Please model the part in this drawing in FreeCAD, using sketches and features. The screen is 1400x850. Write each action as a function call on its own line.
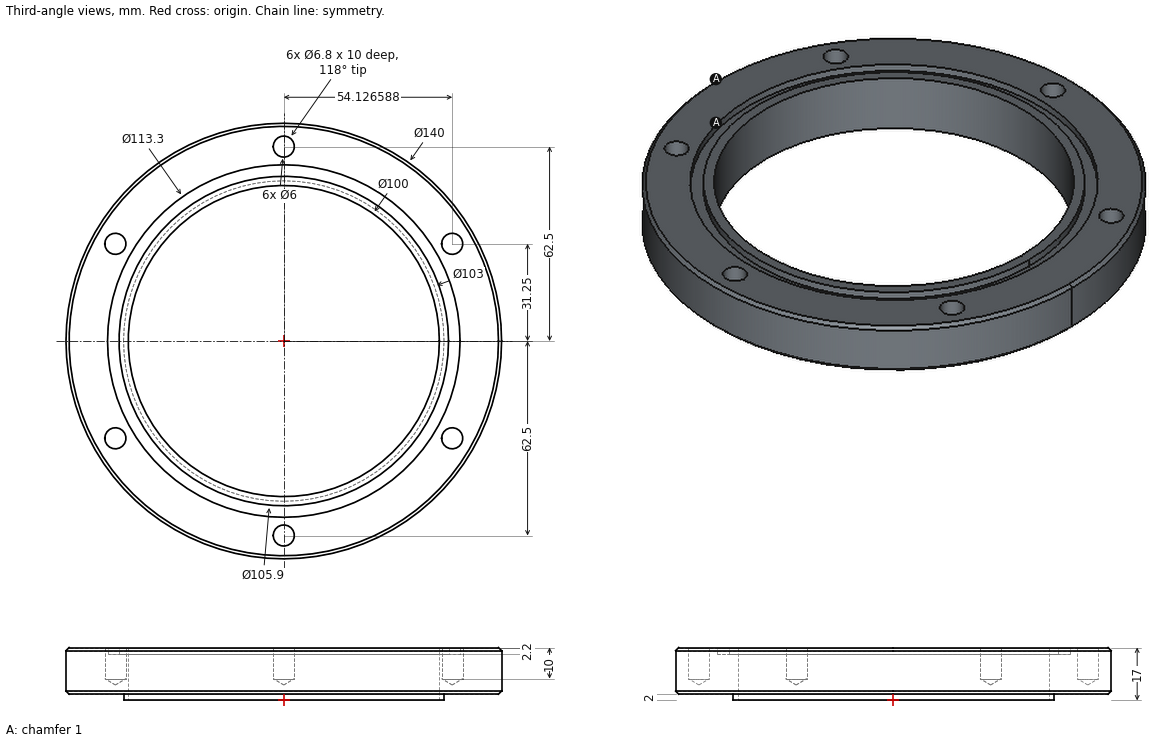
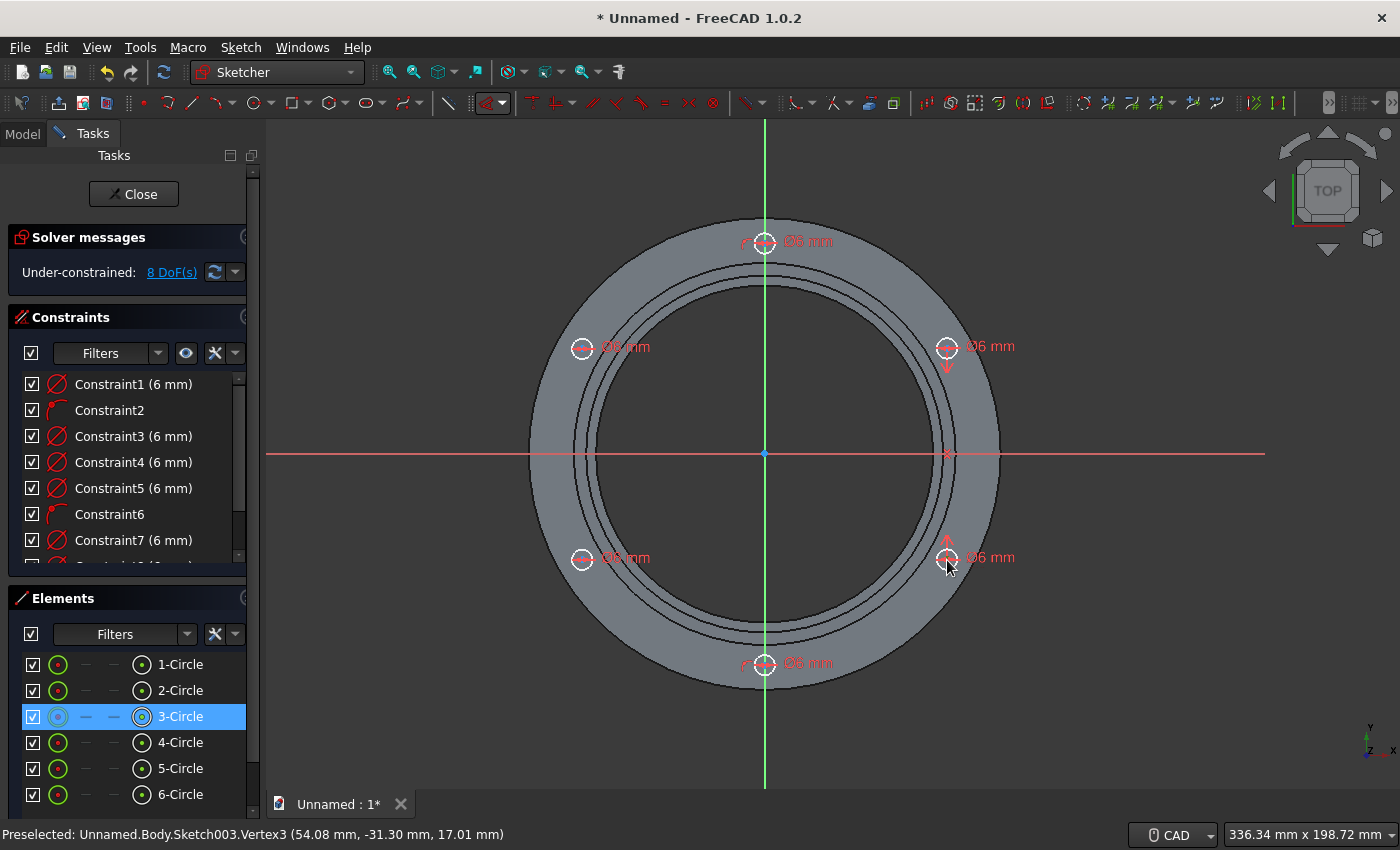
click(582, 560)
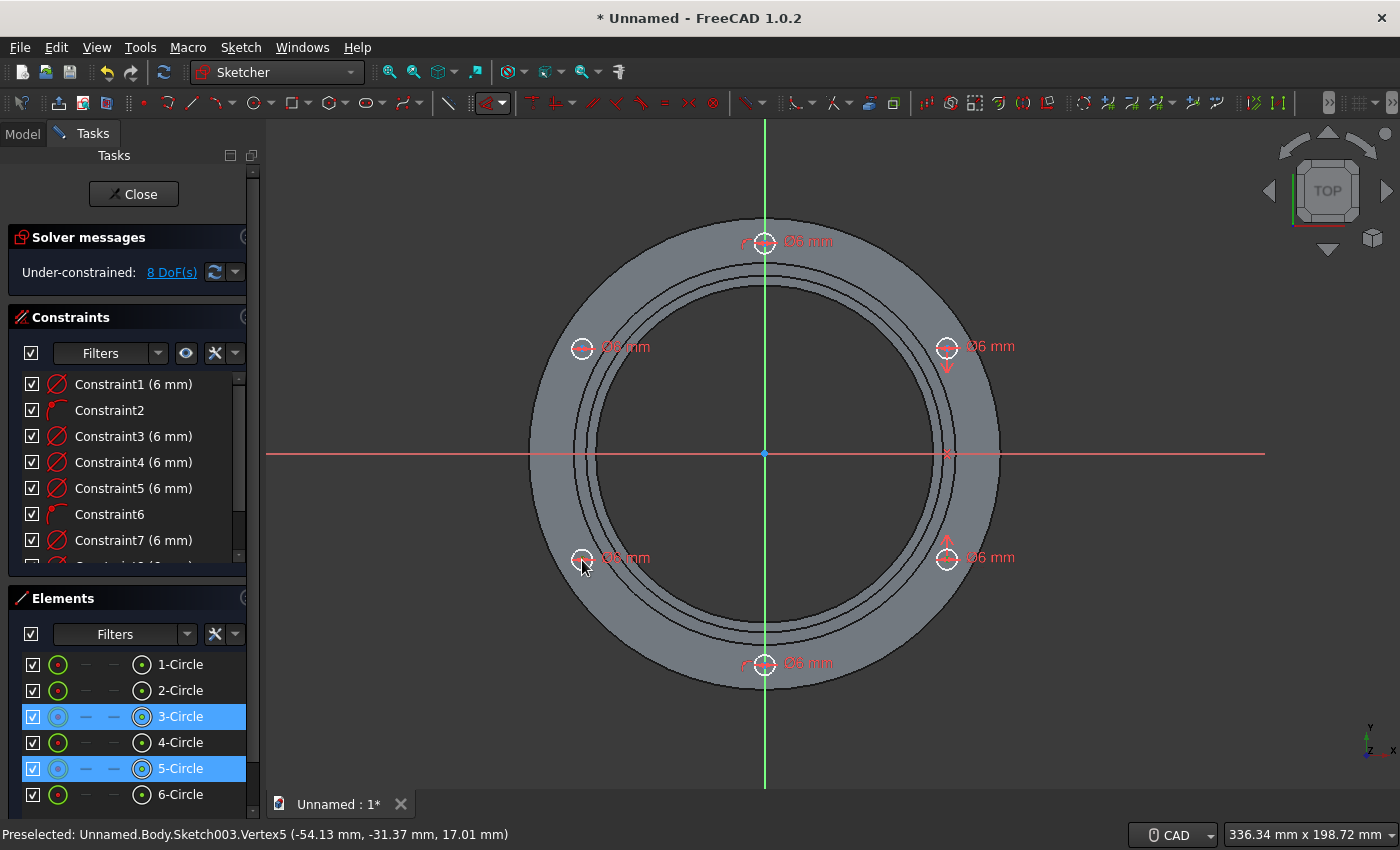
click(765, 717)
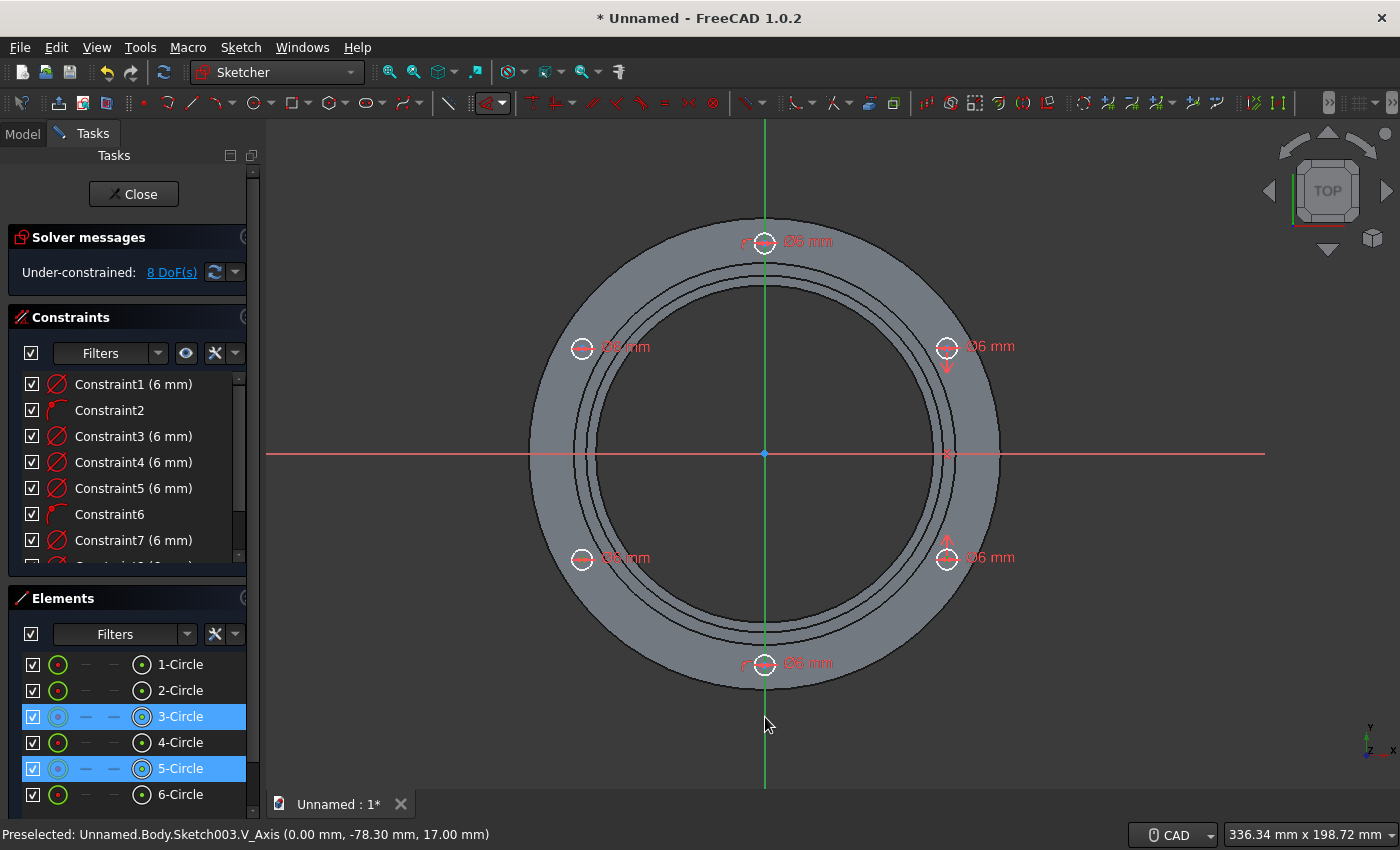
key(s)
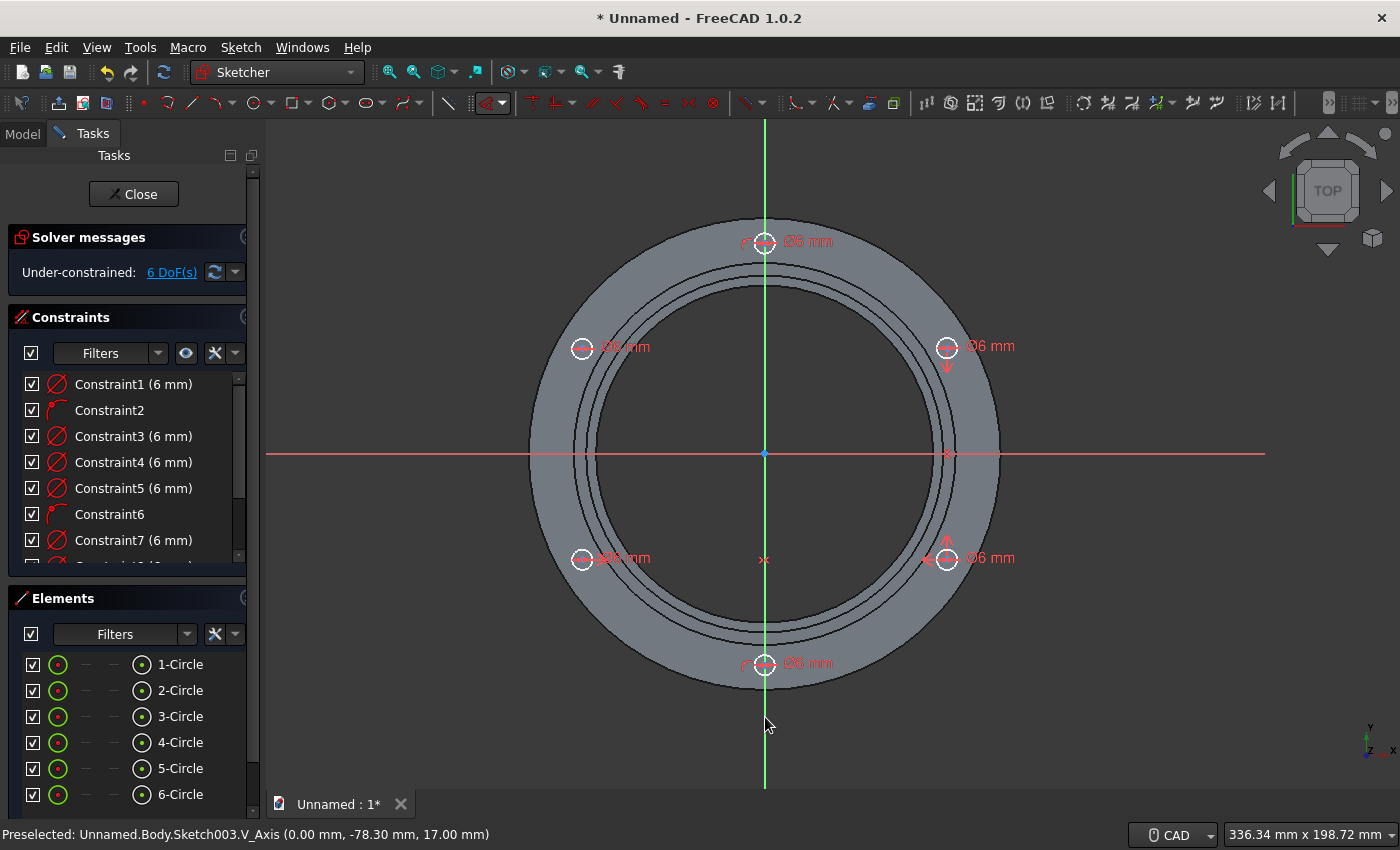
click(947, 348)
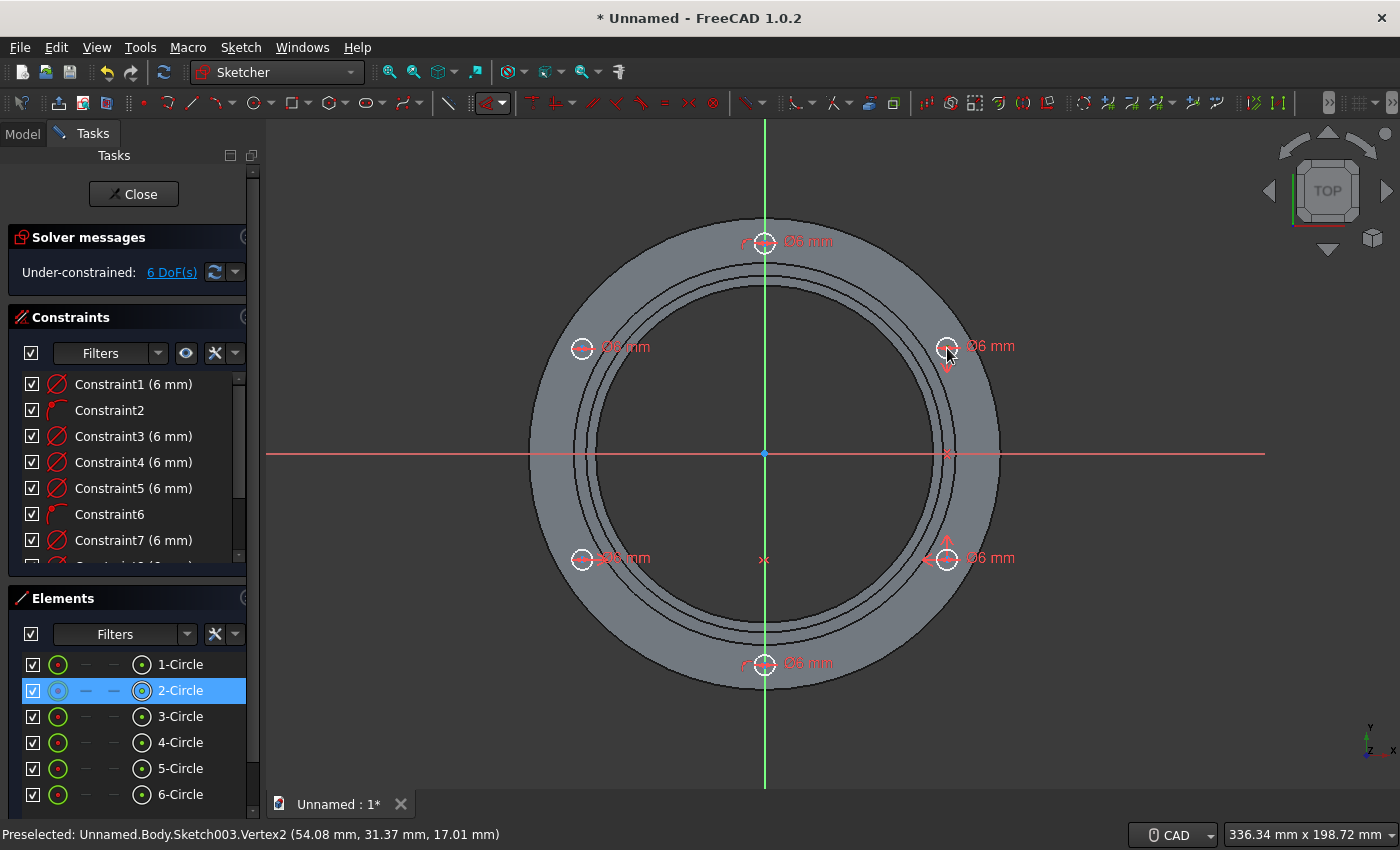
click(582, 349)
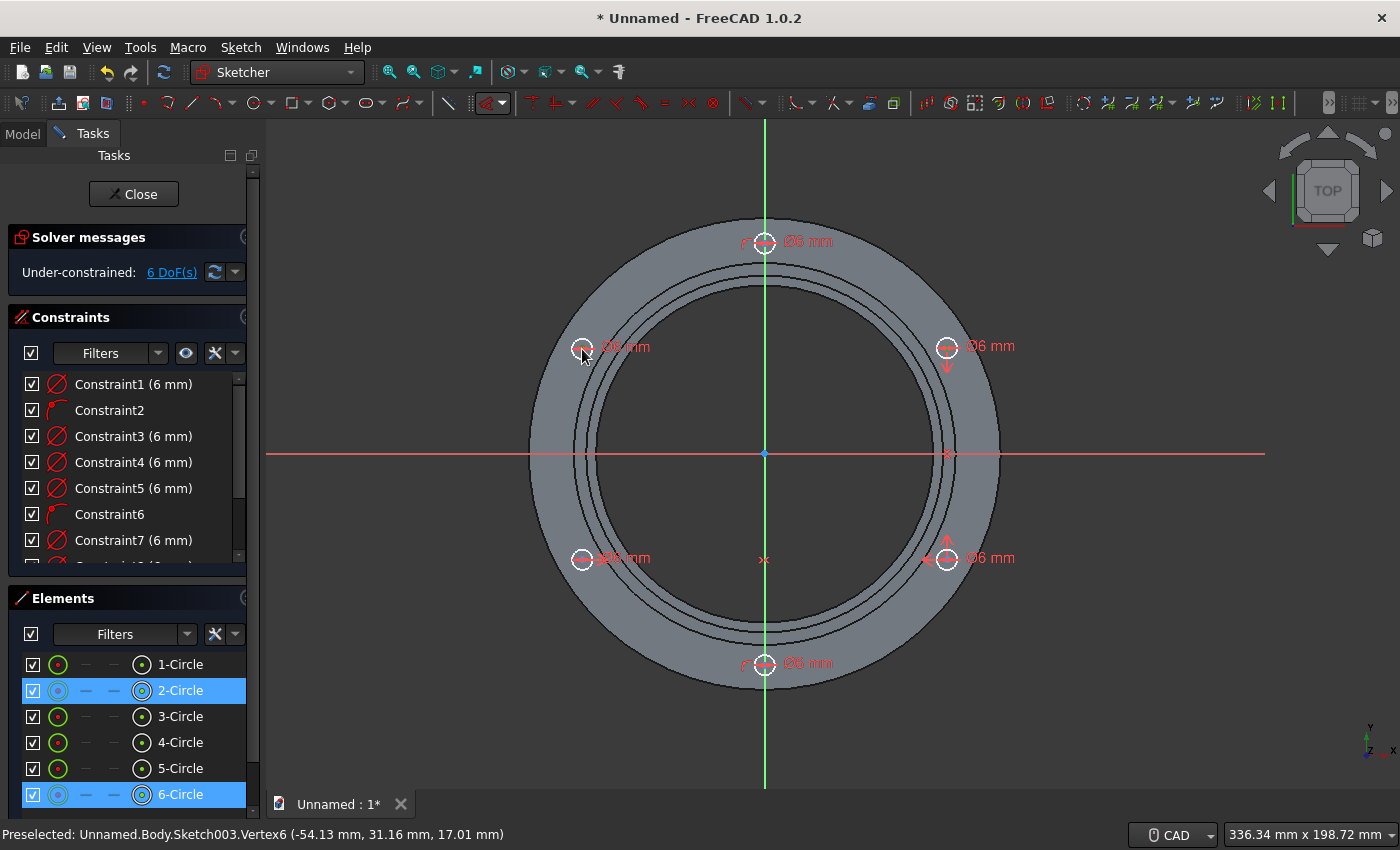
click(765, 717)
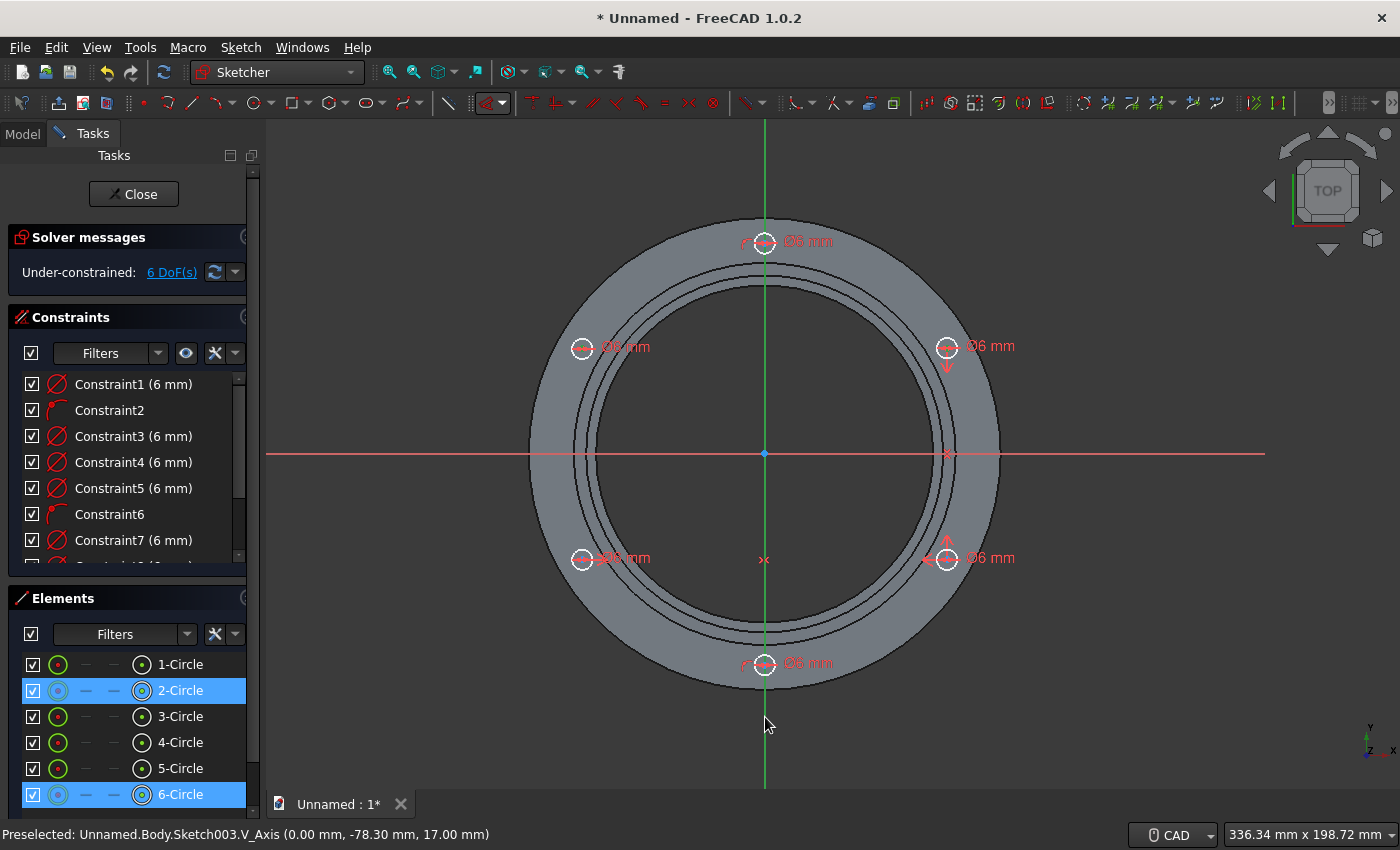
click(690, 104)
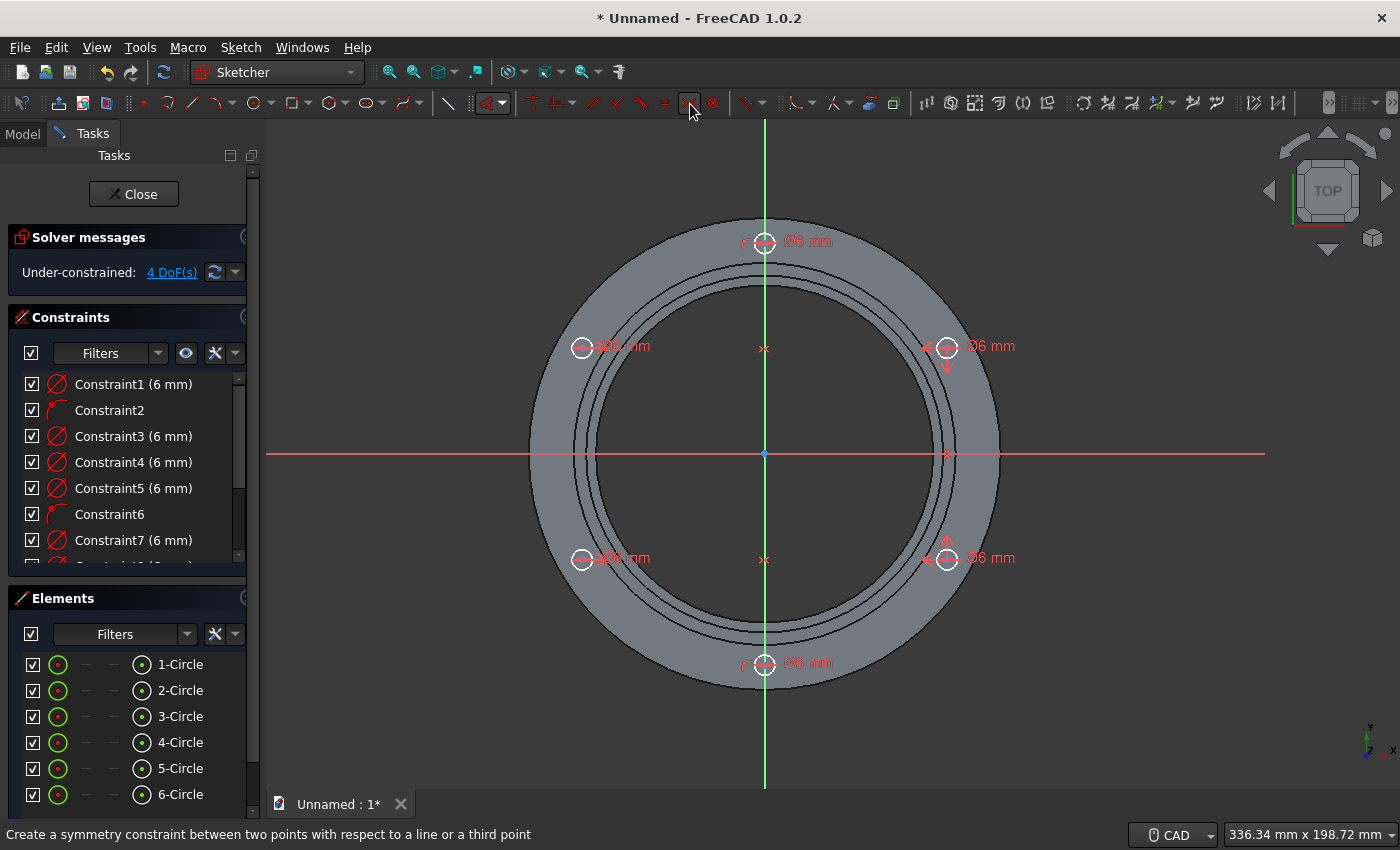
click(765, 243)